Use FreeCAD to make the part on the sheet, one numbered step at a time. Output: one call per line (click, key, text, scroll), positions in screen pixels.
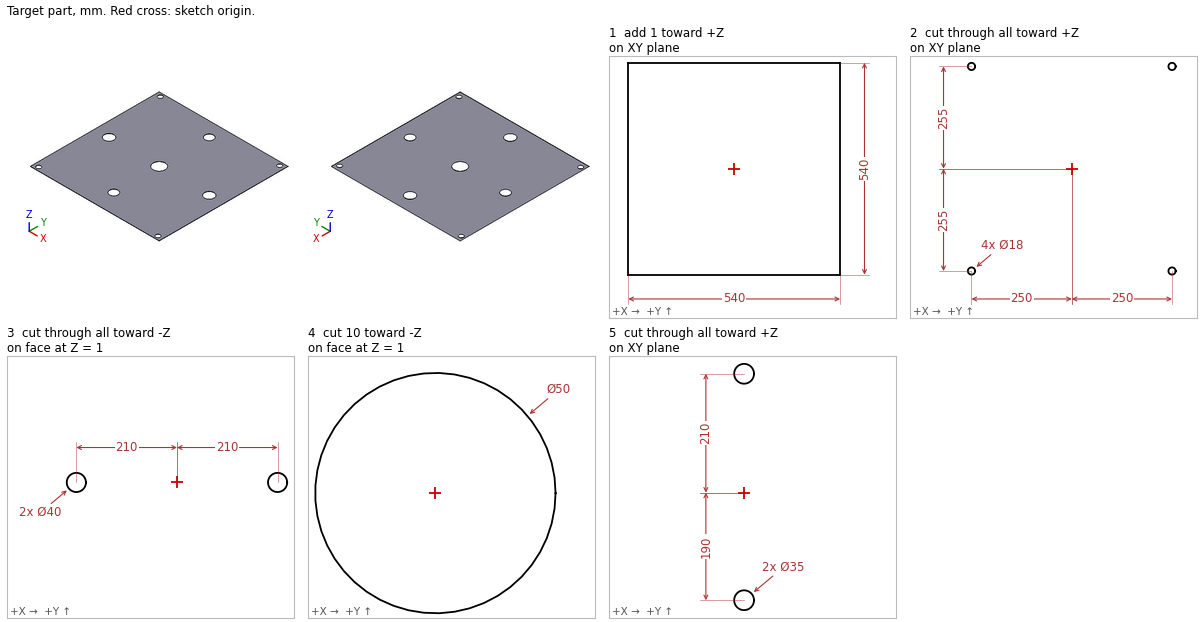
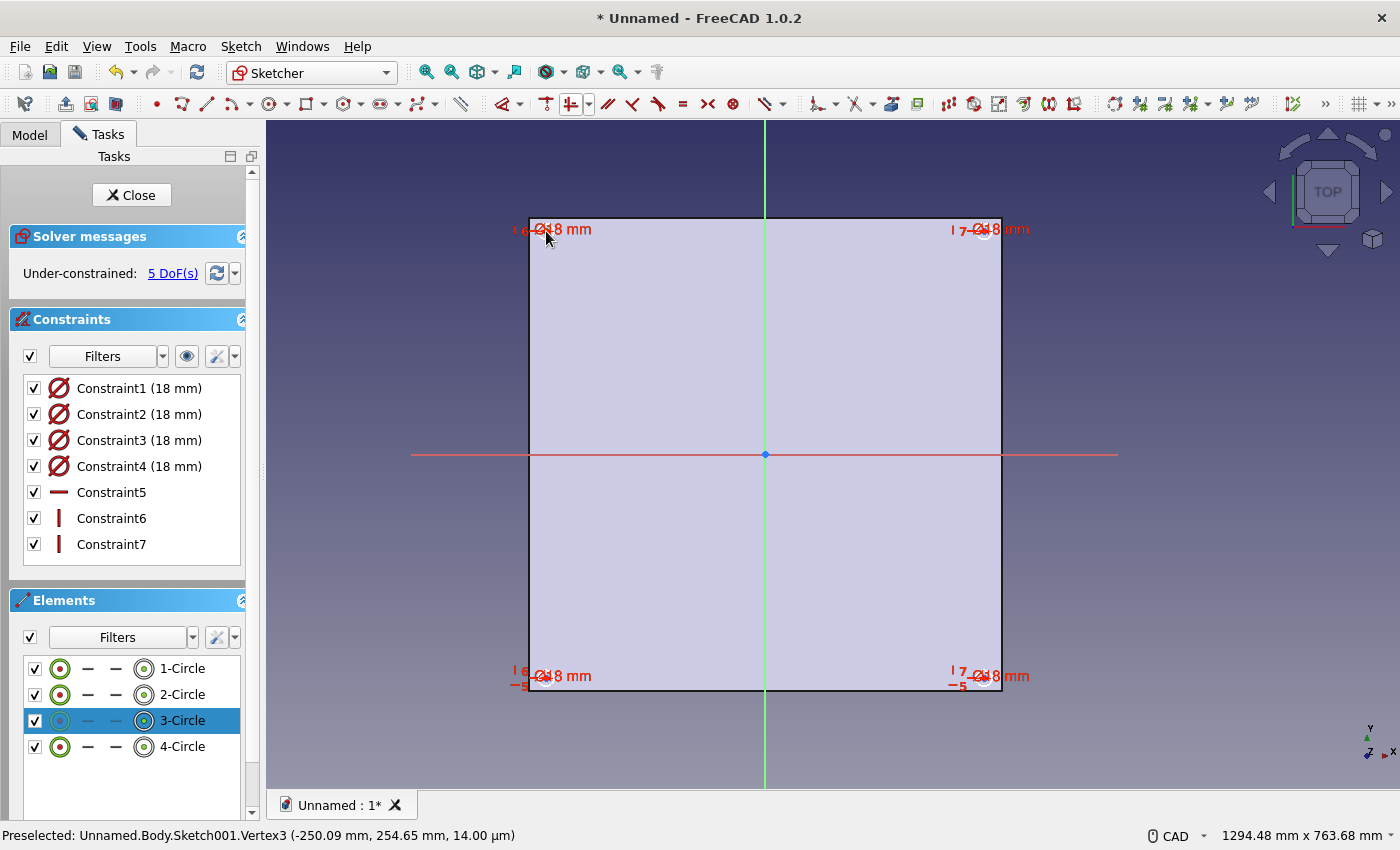
click(984, 231)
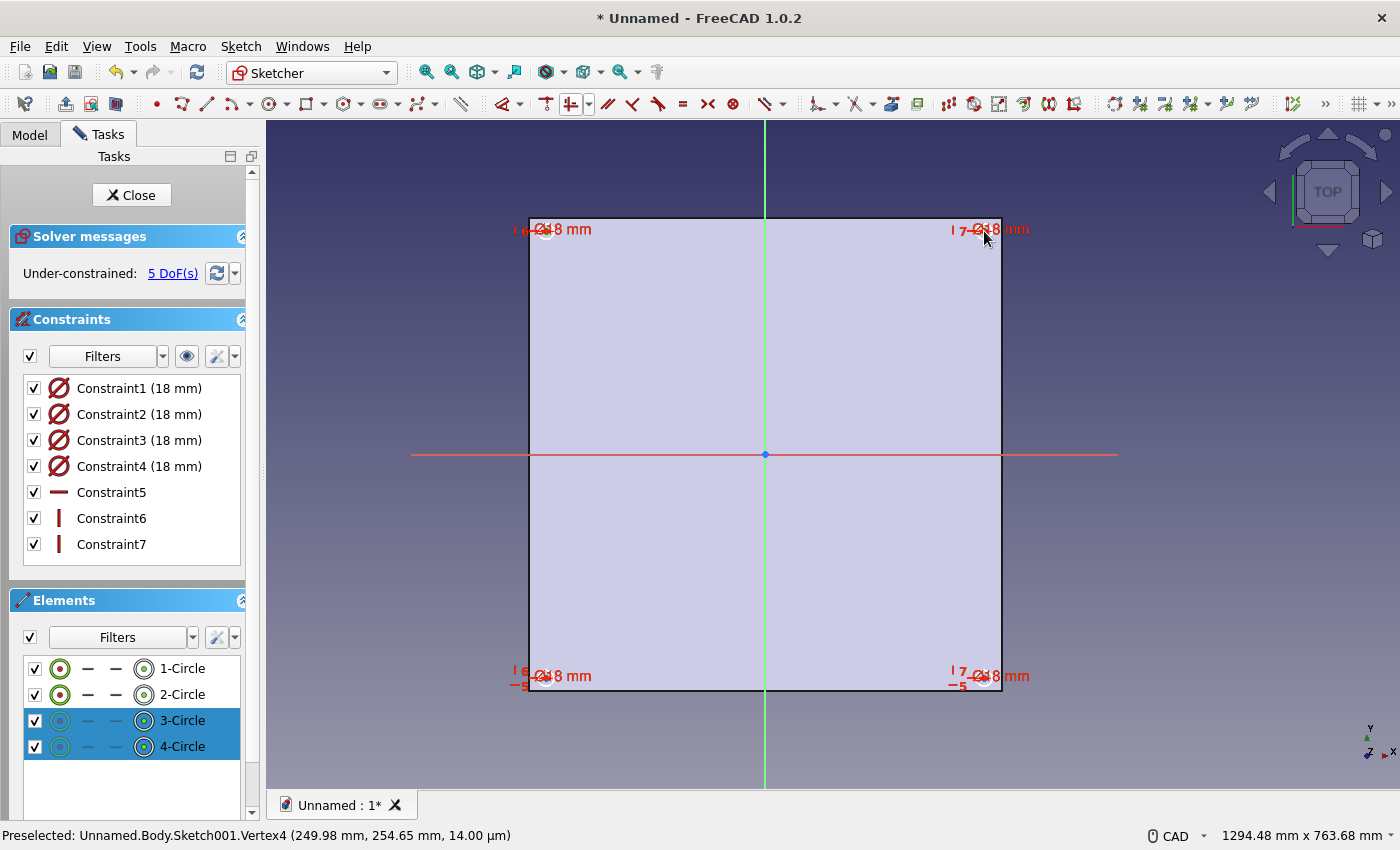
key(h)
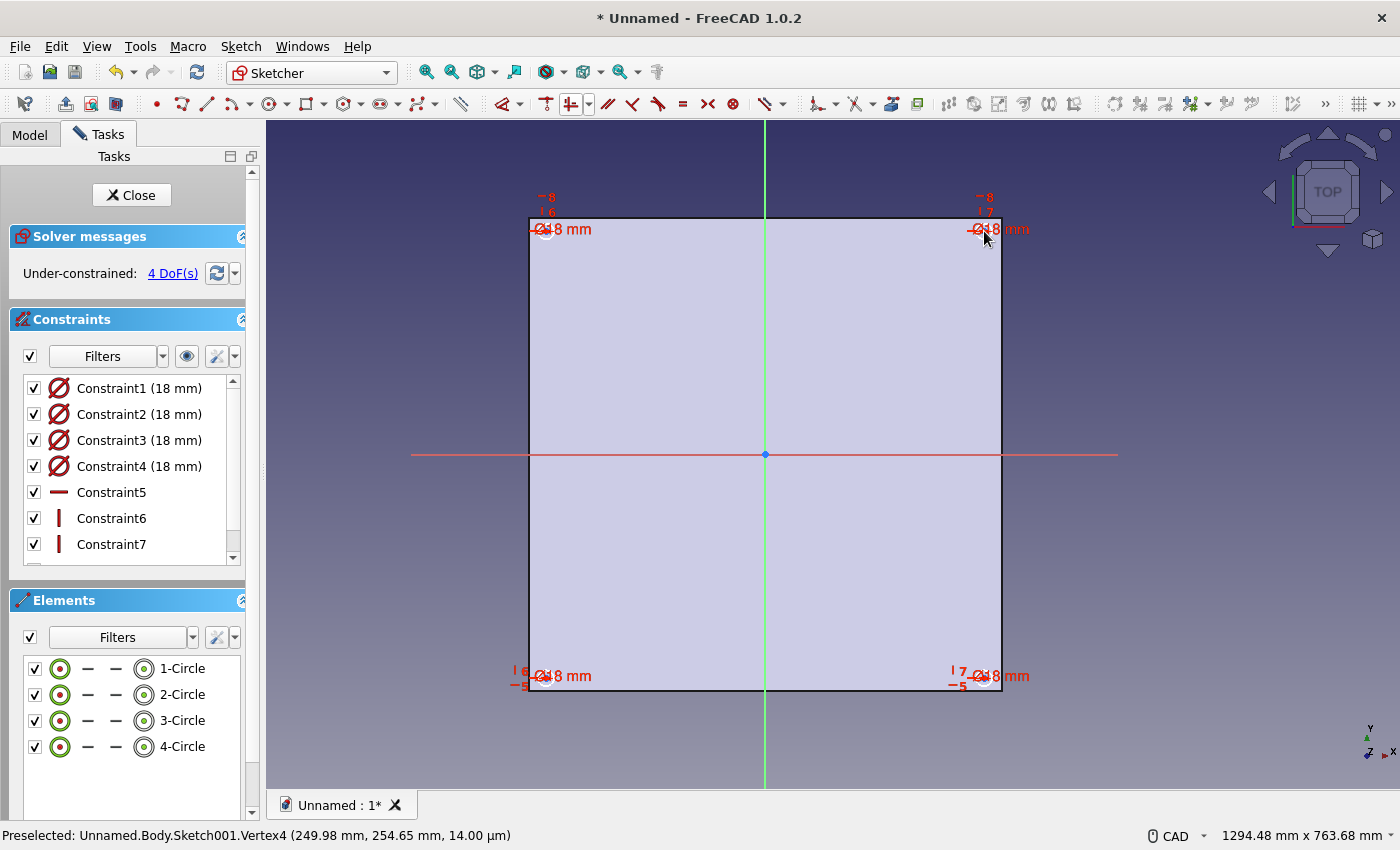
key(d)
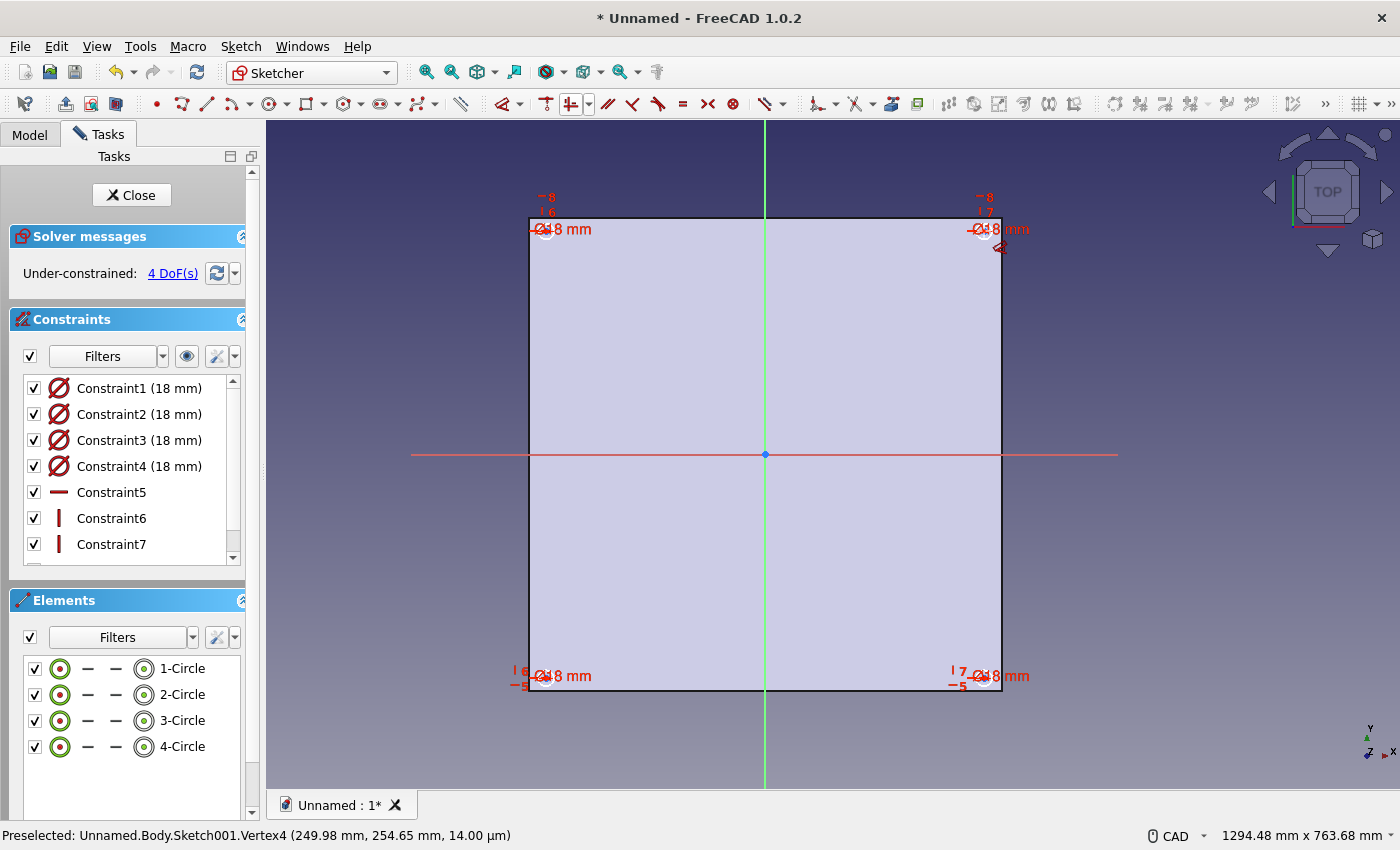
click(546, 678)
click(656, 712)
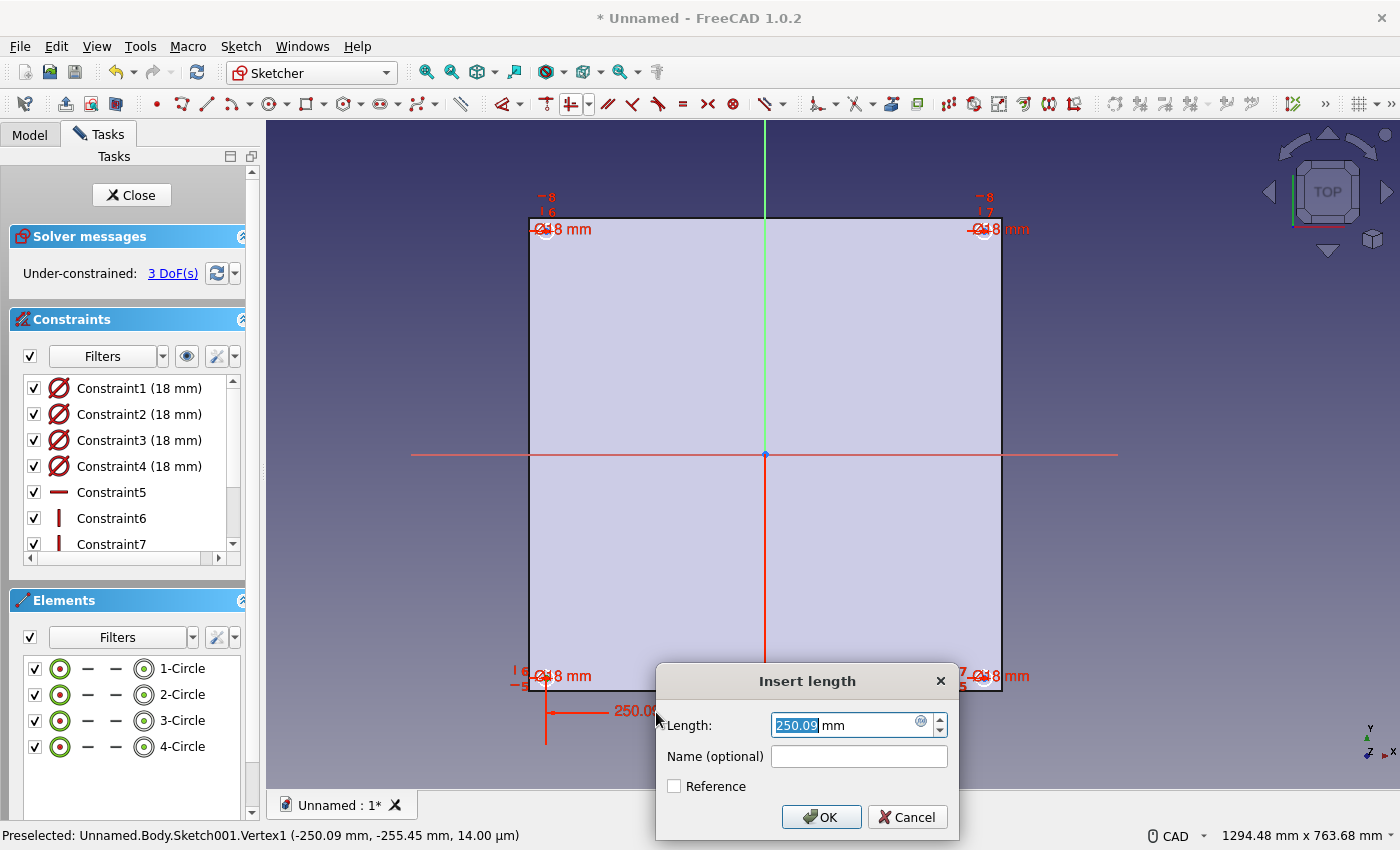
text(250)
key(Return)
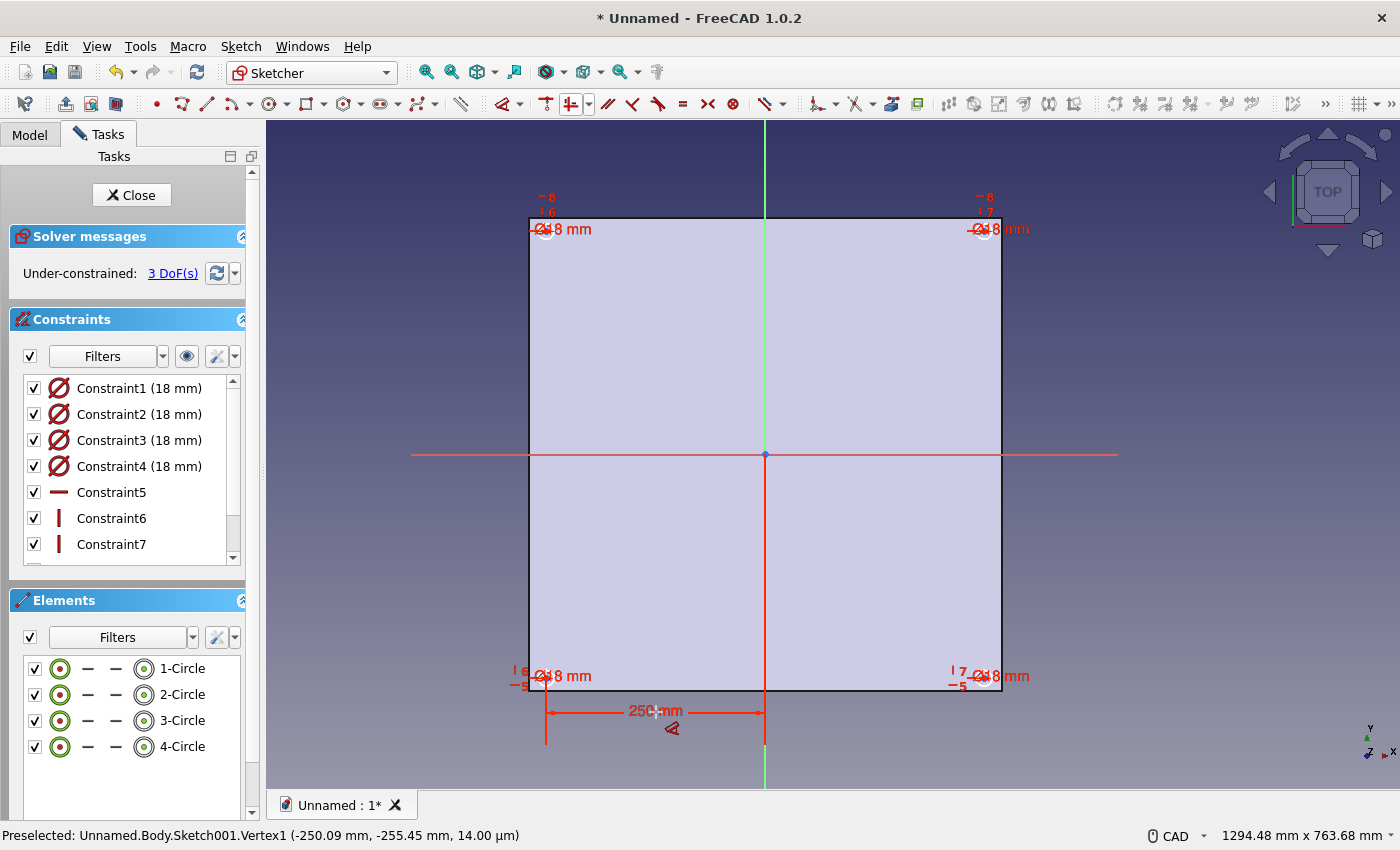
click(546, 678)
click(512, 566)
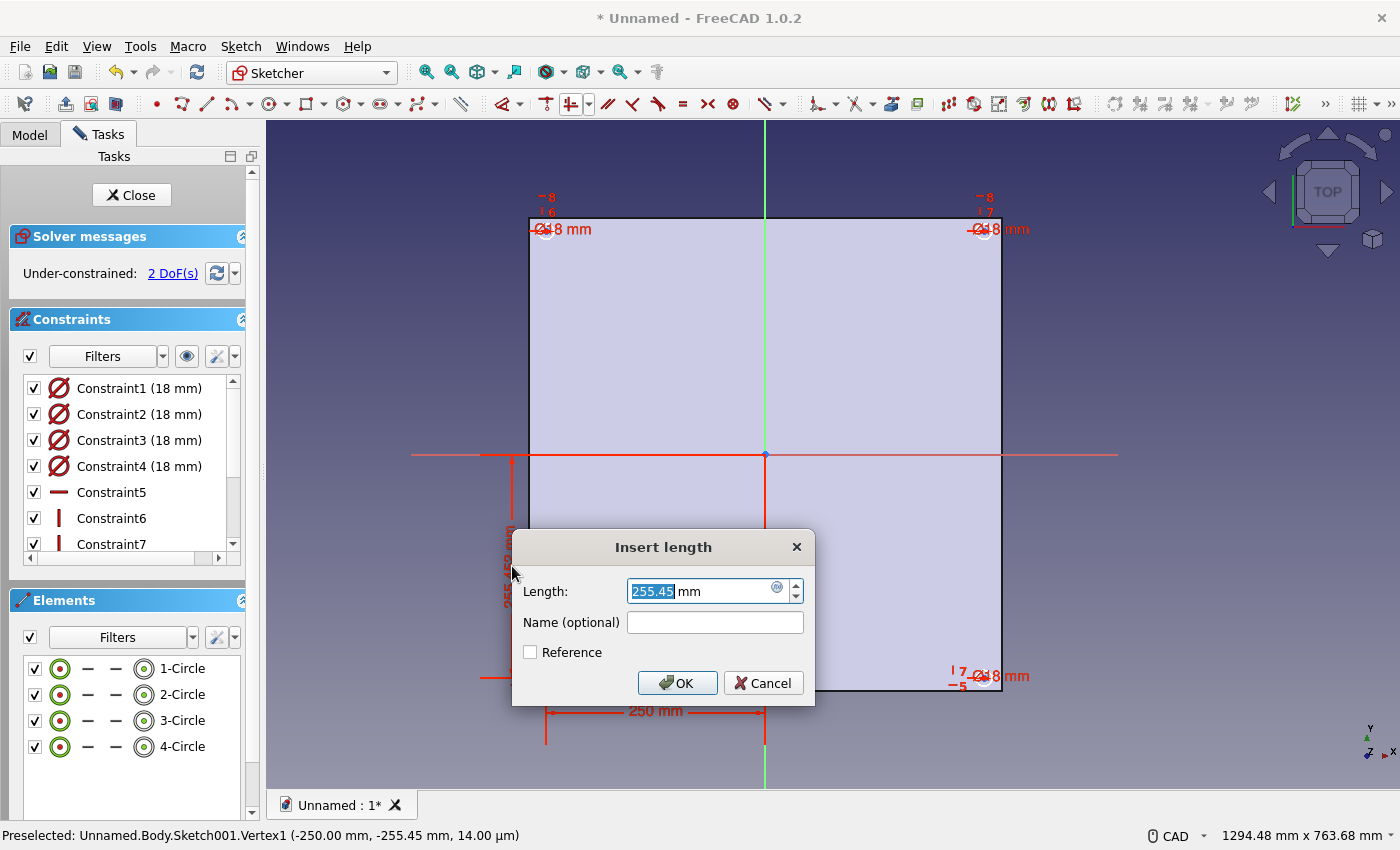
text(255)
key(Return)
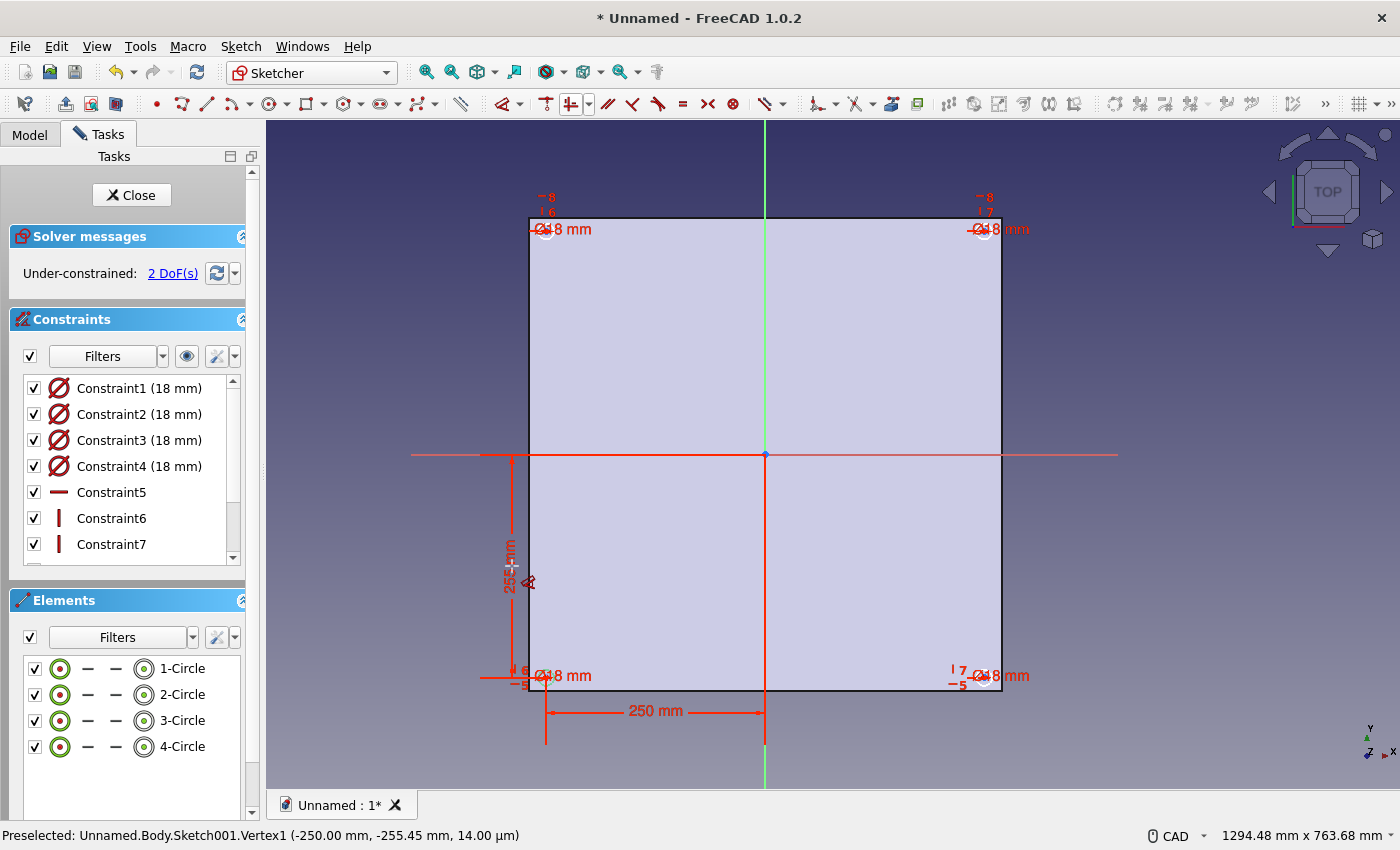
click(984, 678)
click(875, 712)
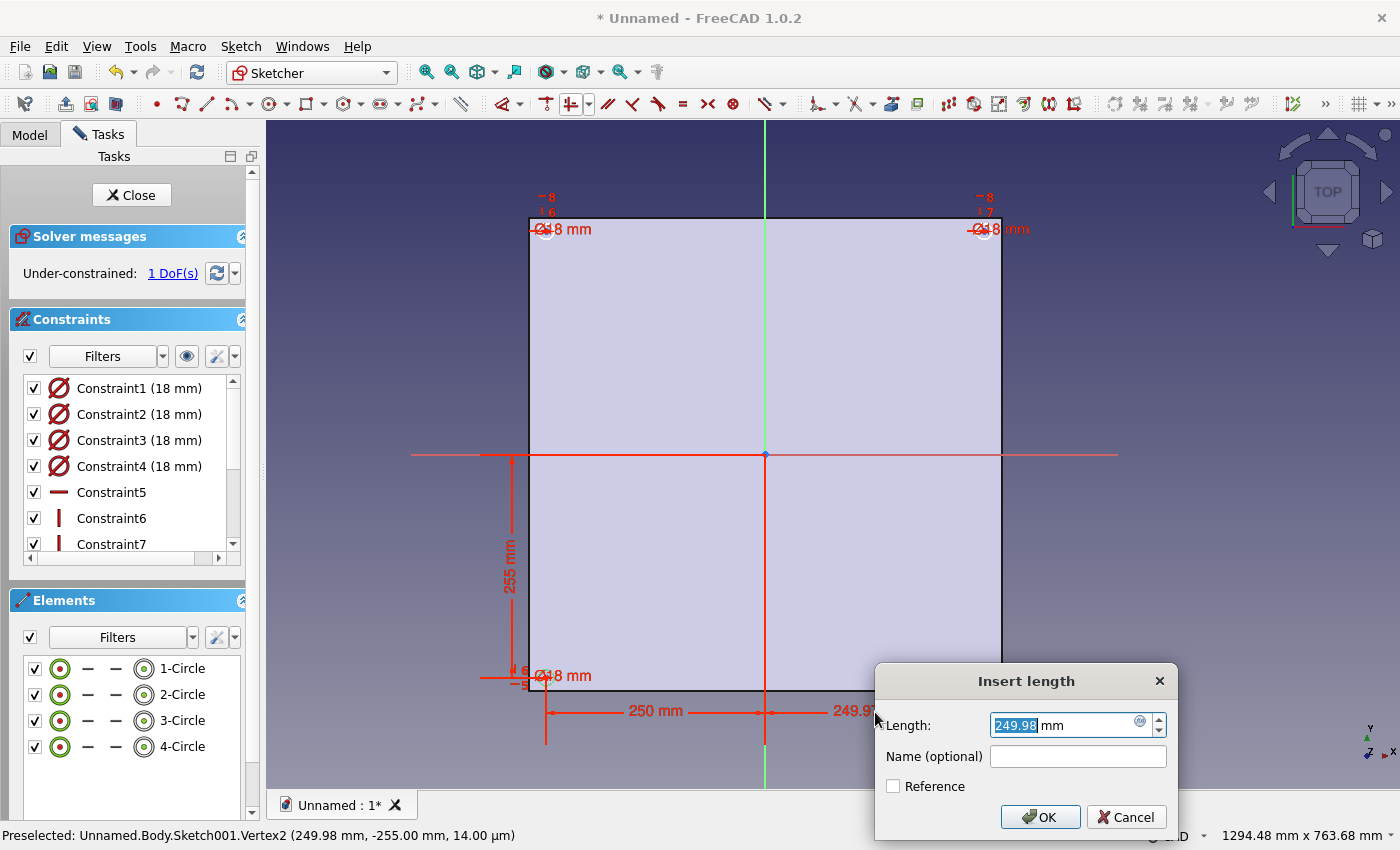
text(250)
key(Return)